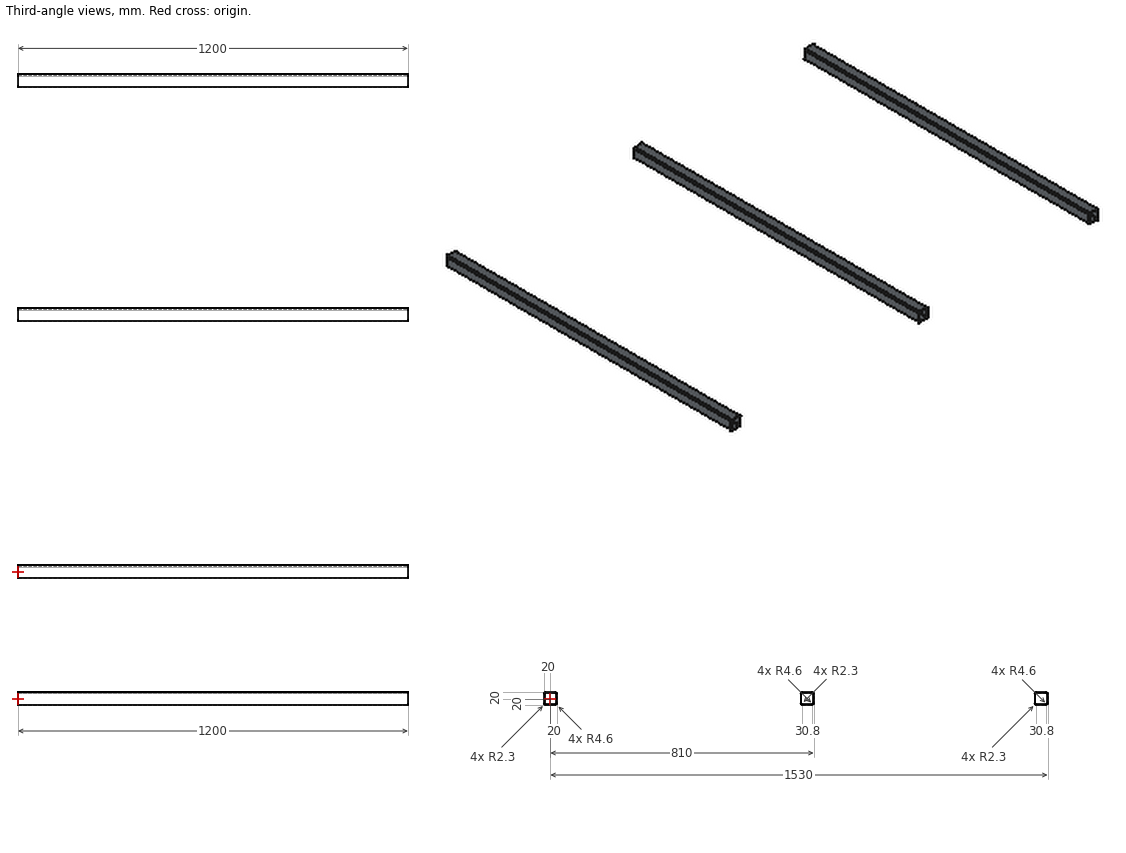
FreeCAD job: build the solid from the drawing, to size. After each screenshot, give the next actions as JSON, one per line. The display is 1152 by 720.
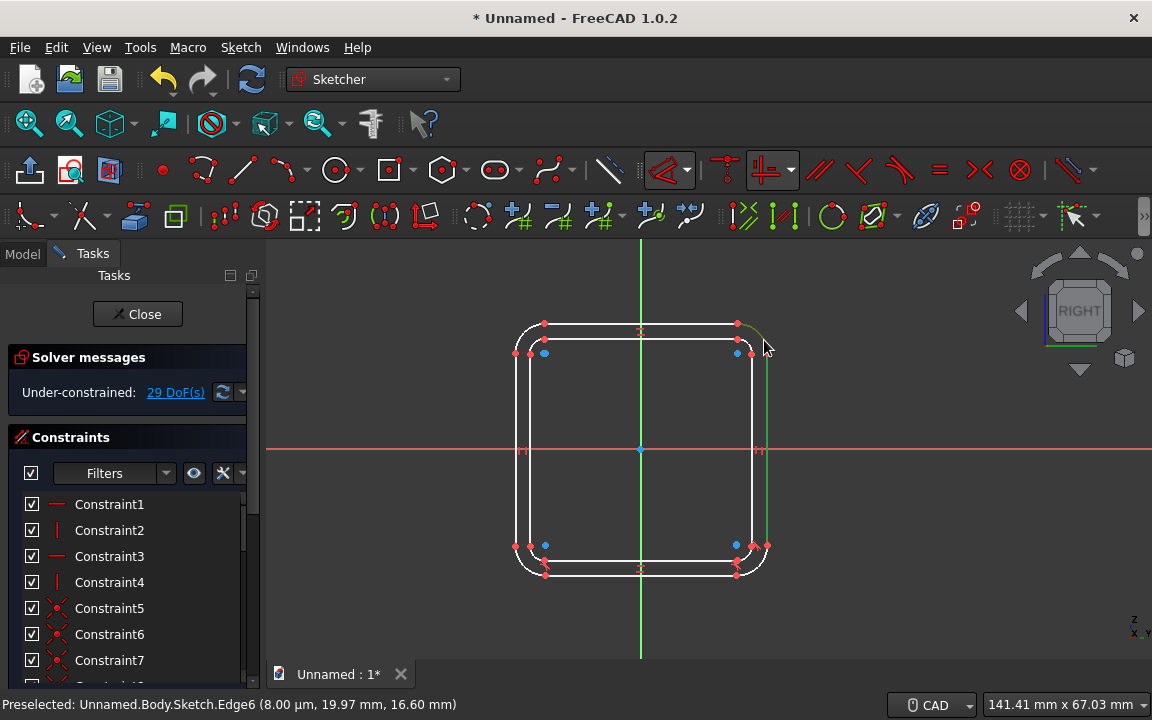
{"action": "key", "text": "t"}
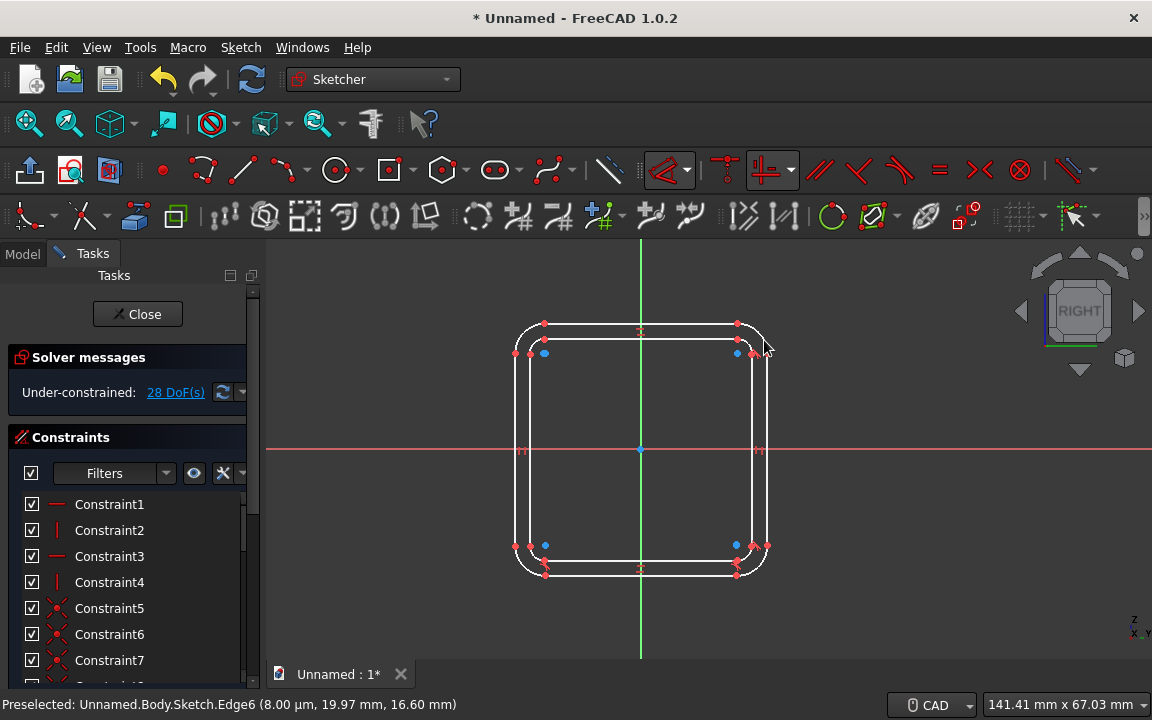
{"action": "left_click", "coordinate": [680, 324]}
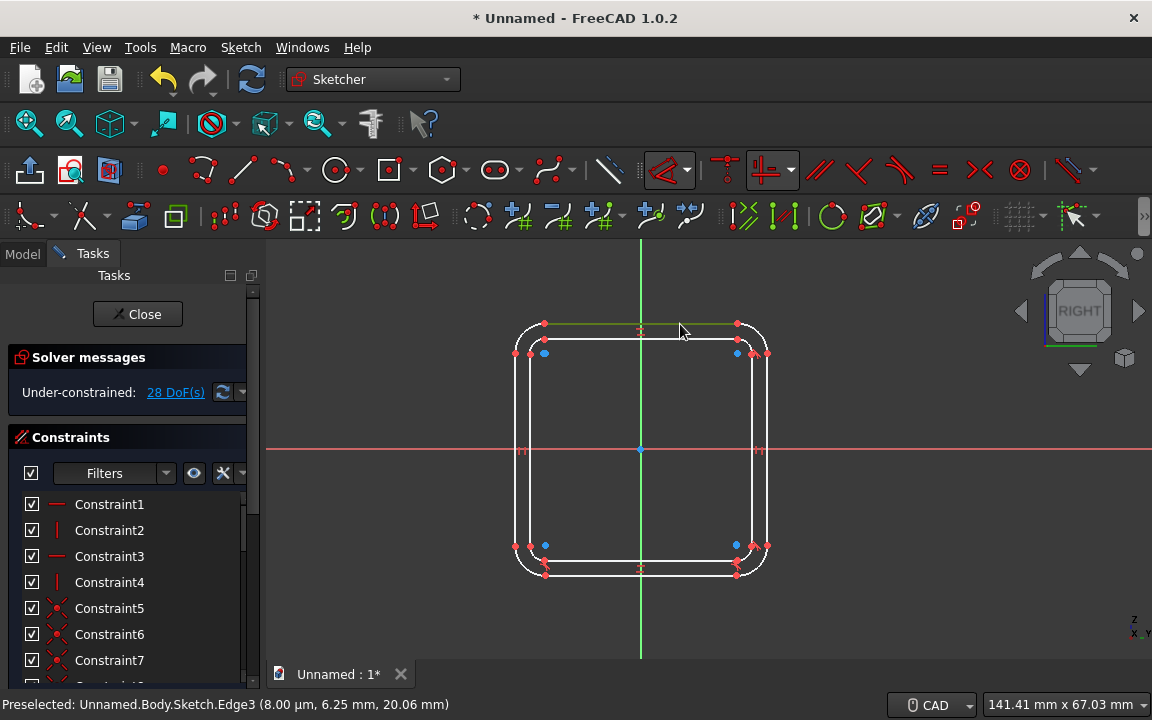
{"action": "left_click", "coordinate": [764, 340]}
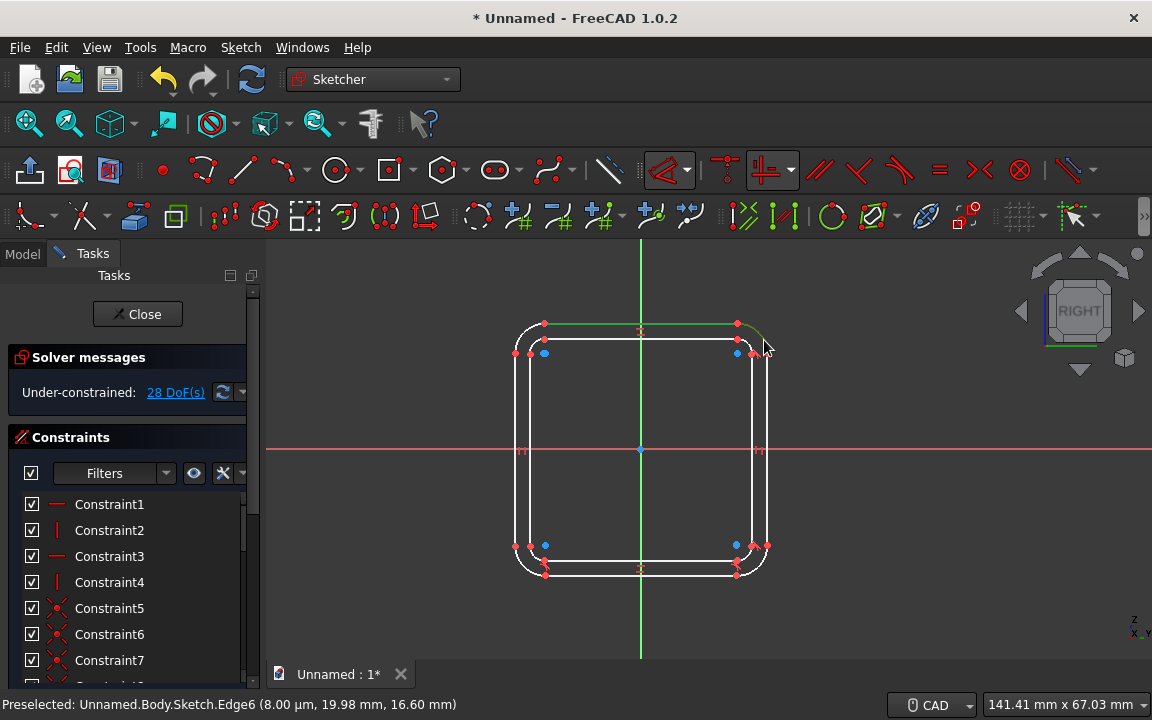
{"action": "key", "text": "t"}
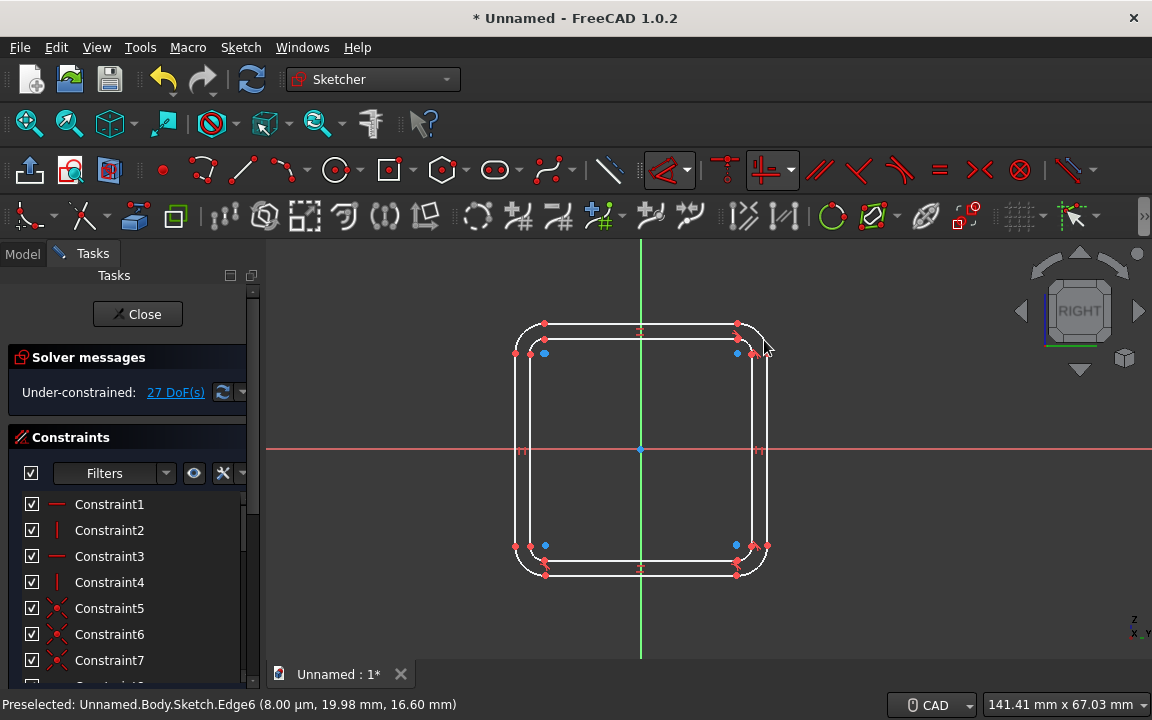
{"action": "left_click", "coordinate": [679, 324]}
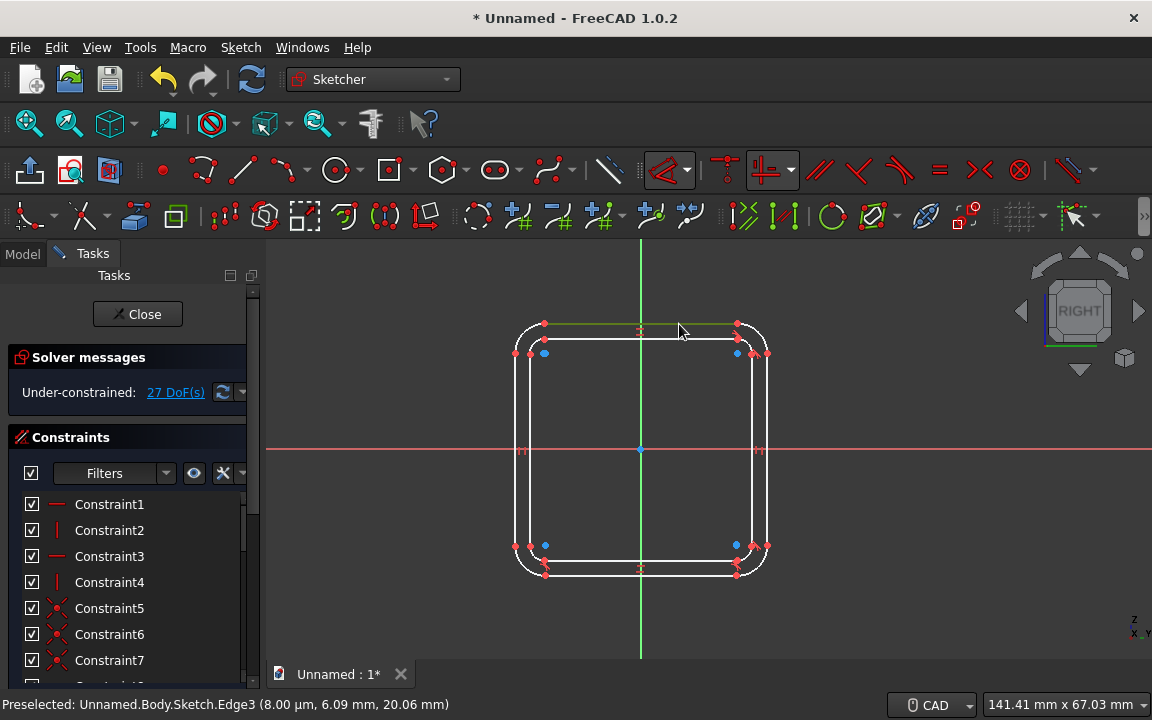
{"action": "left_click", "coordinate": [531, 327]}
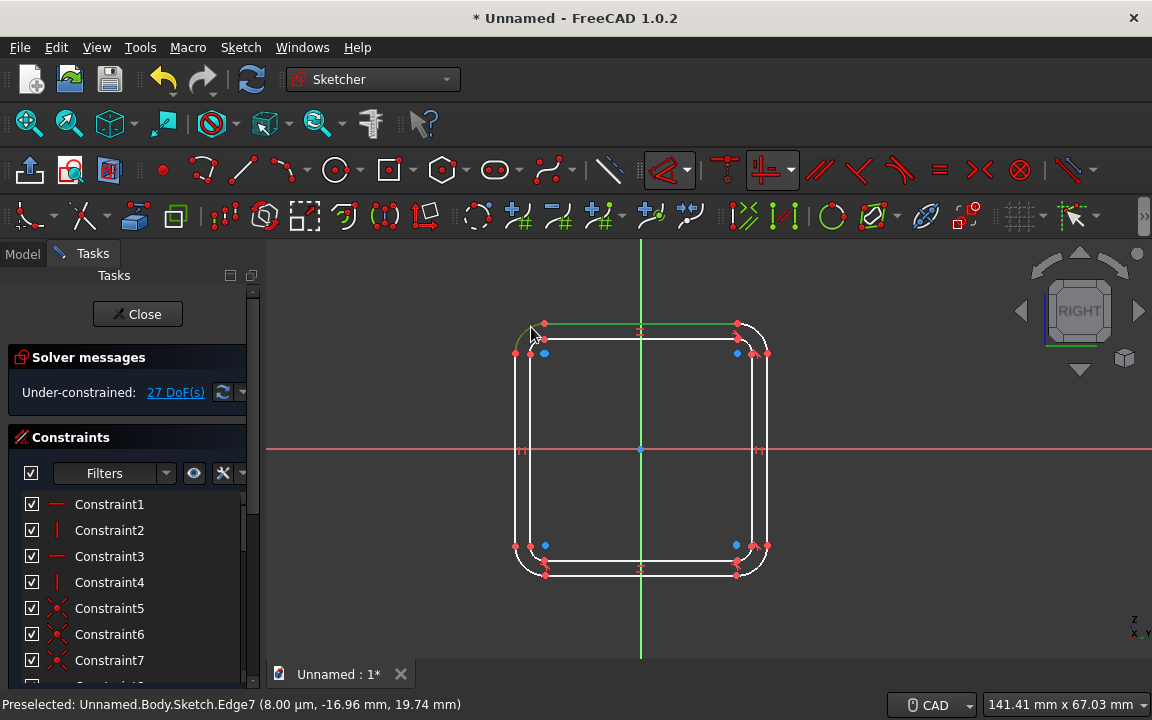
{"action": "left_click", "coordinate": [900, 170]}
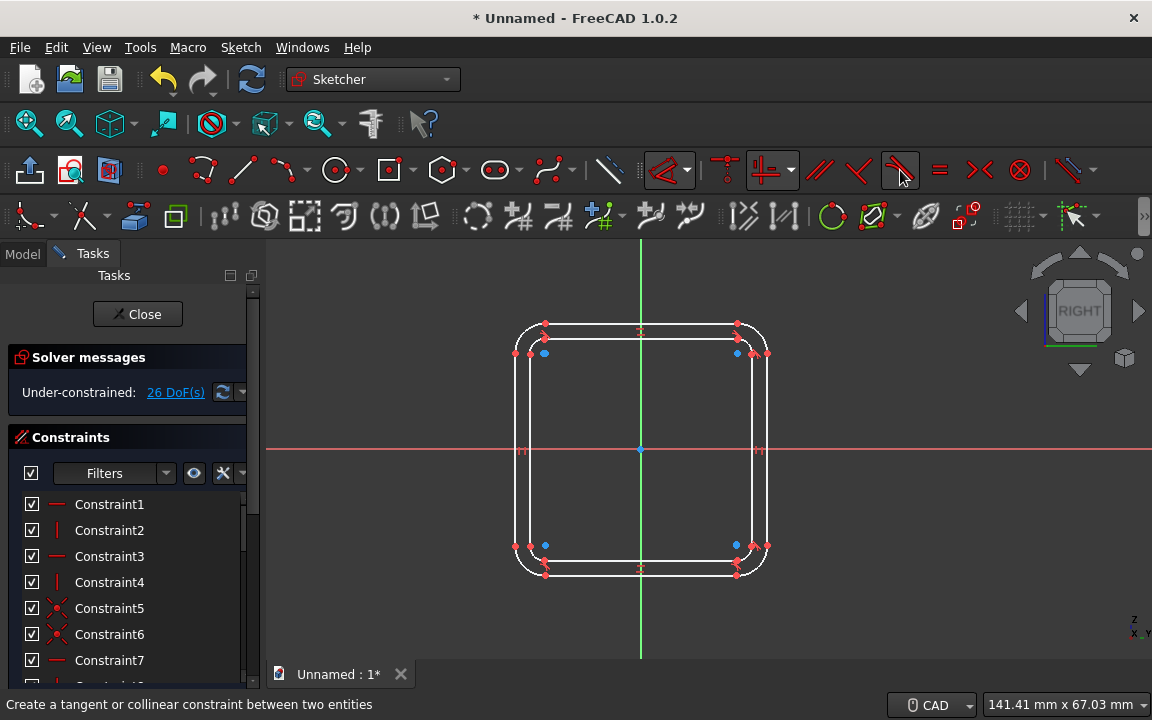
{"action": "left_click", "coordinate": [515, 411]}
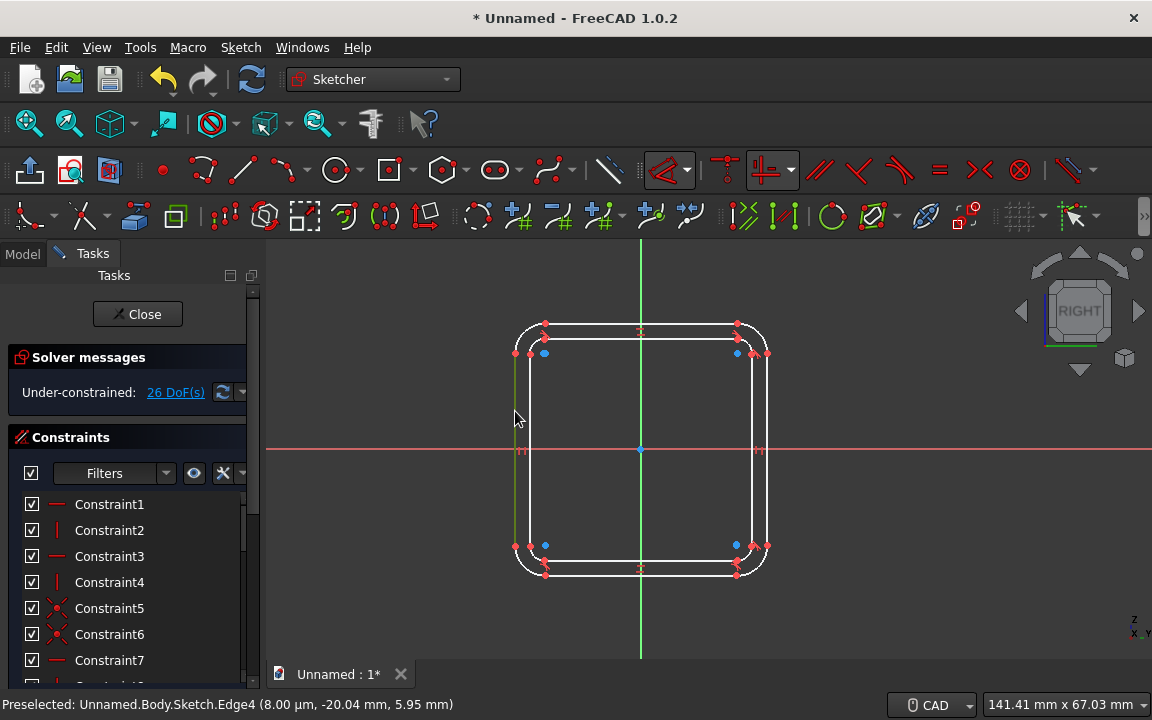
{"action": "left_click", "coordinate": [532, 327]}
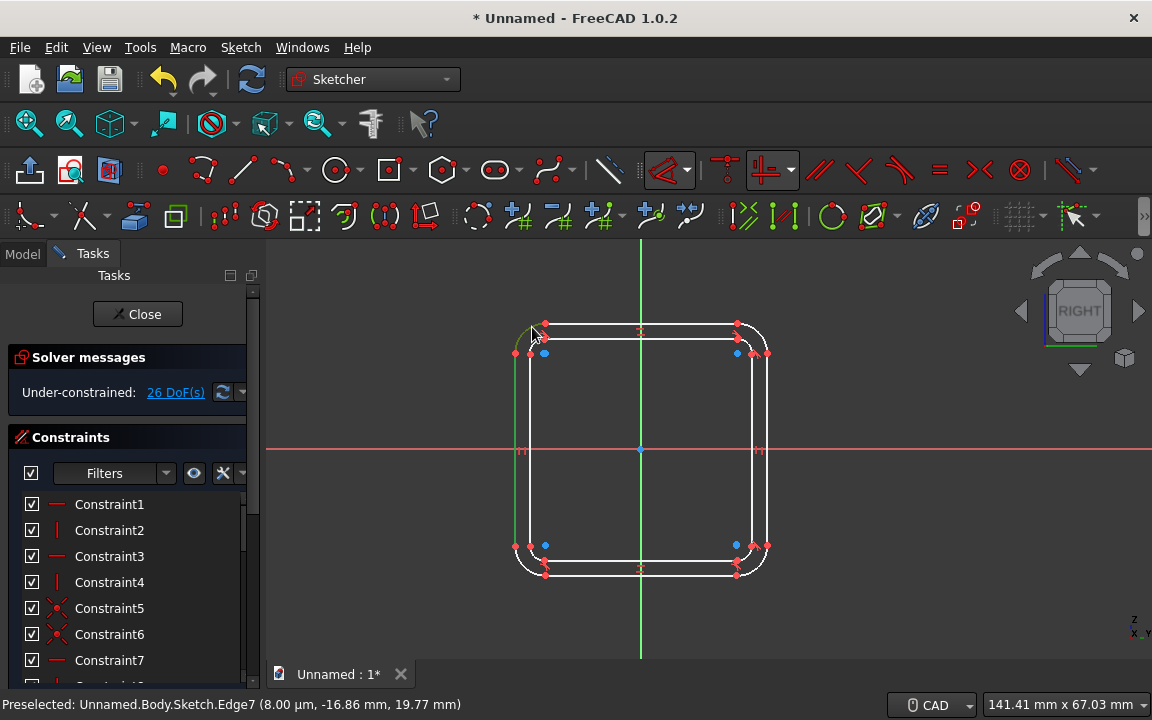
{"action": "left_click", "coordinate": [900, 170]}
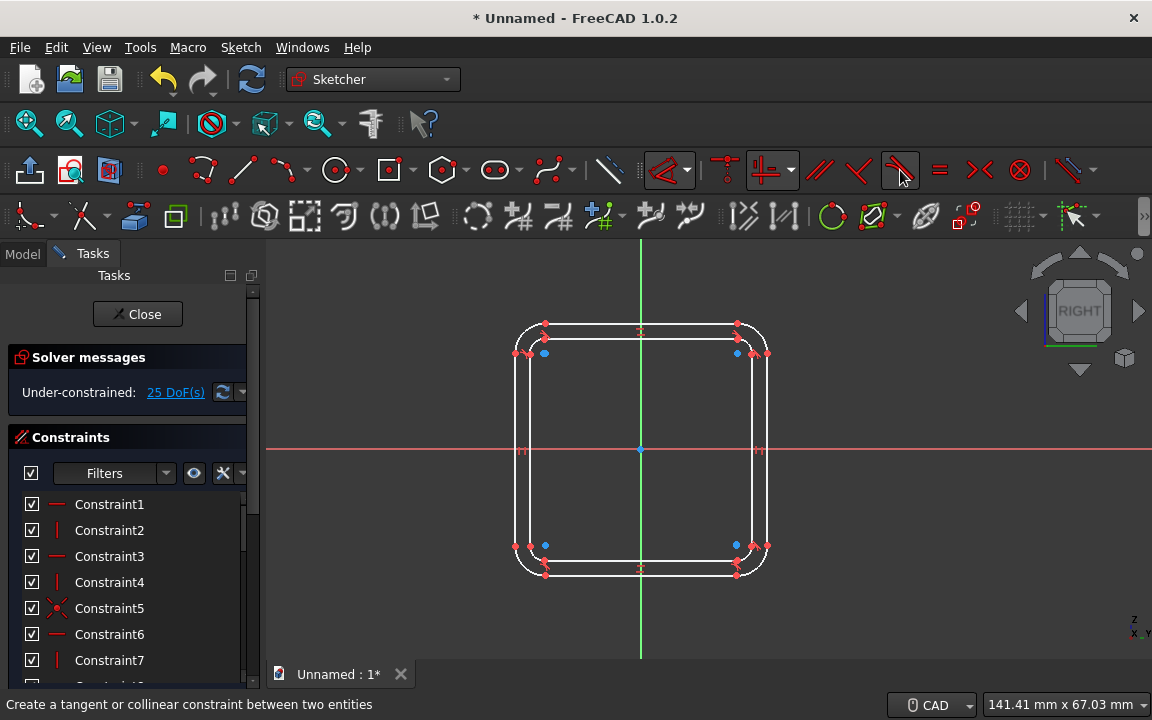
{"action": "left_click", "coordinate": [515, 412]}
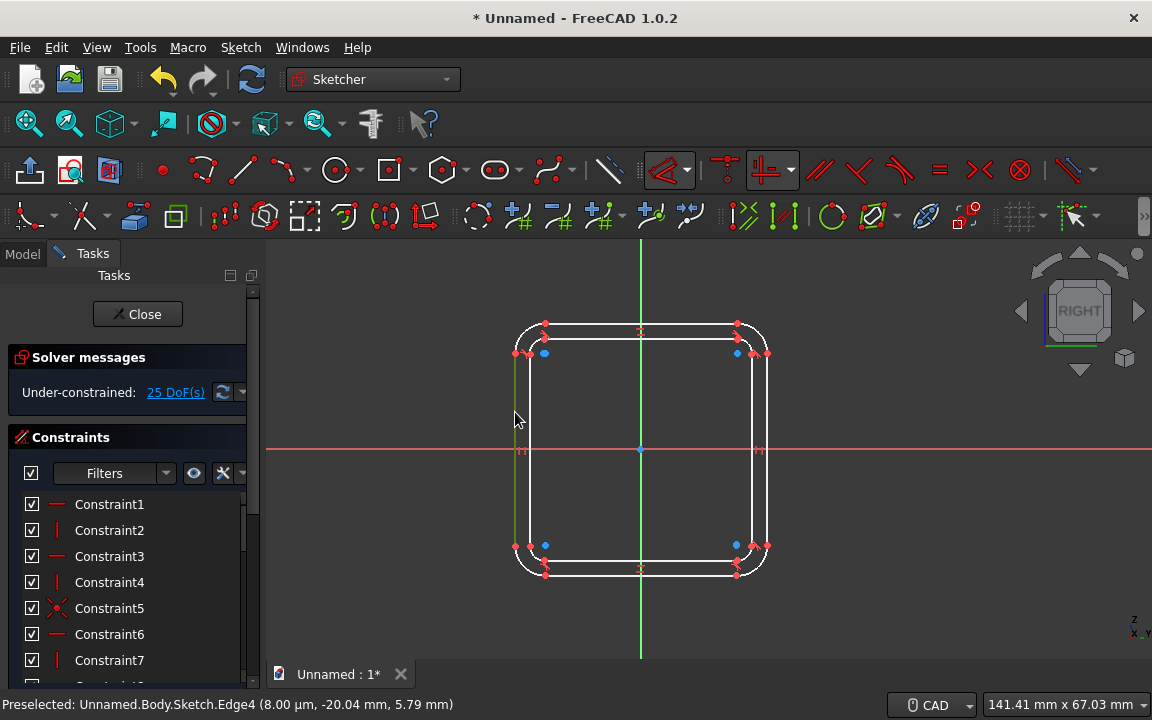
{"action": "left_click", "coordinate": [519, 560]}